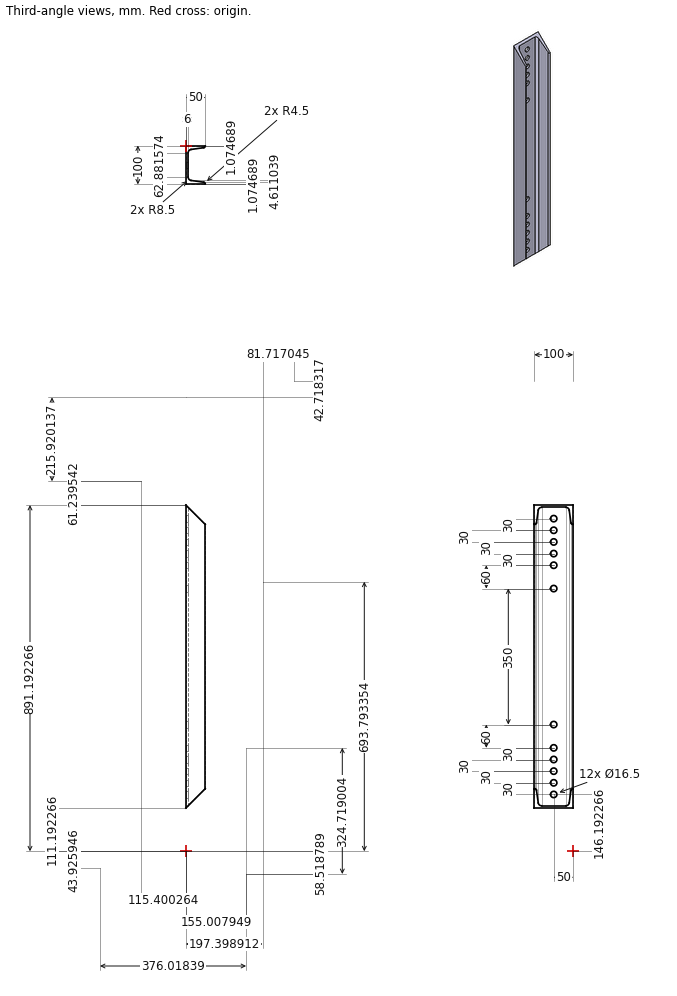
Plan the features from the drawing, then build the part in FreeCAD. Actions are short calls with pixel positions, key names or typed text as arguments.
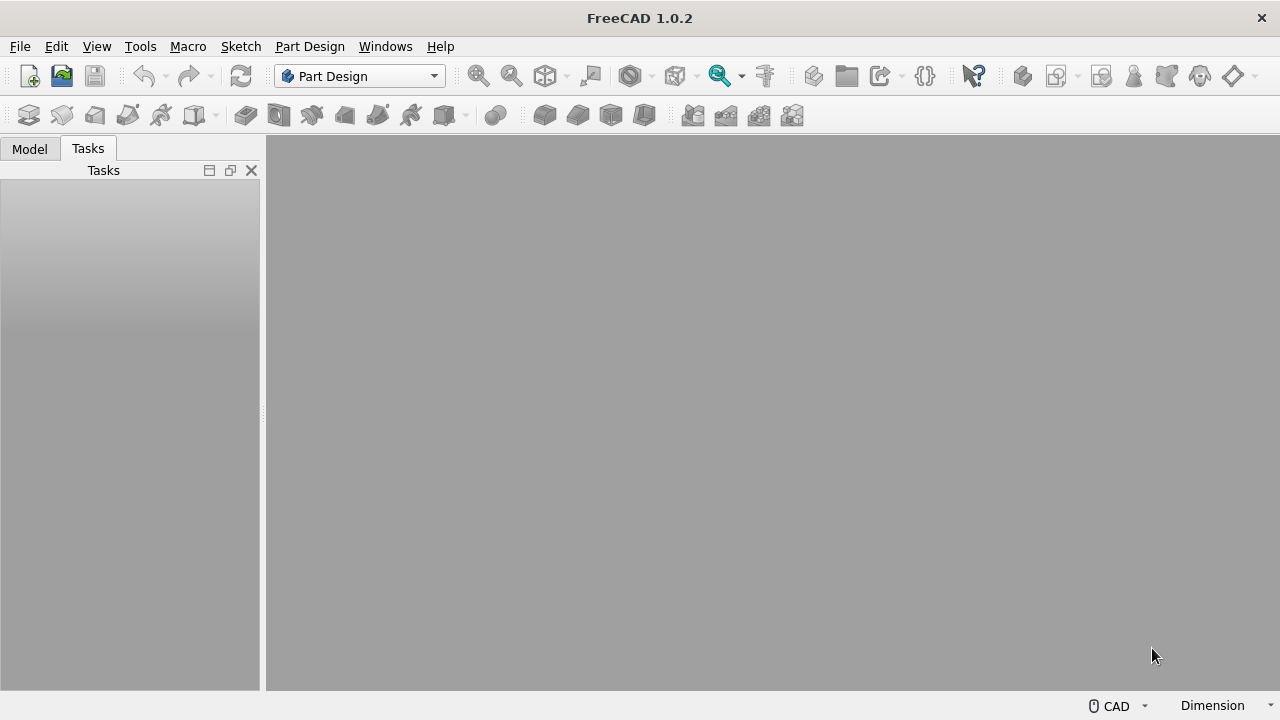
click(29, 76)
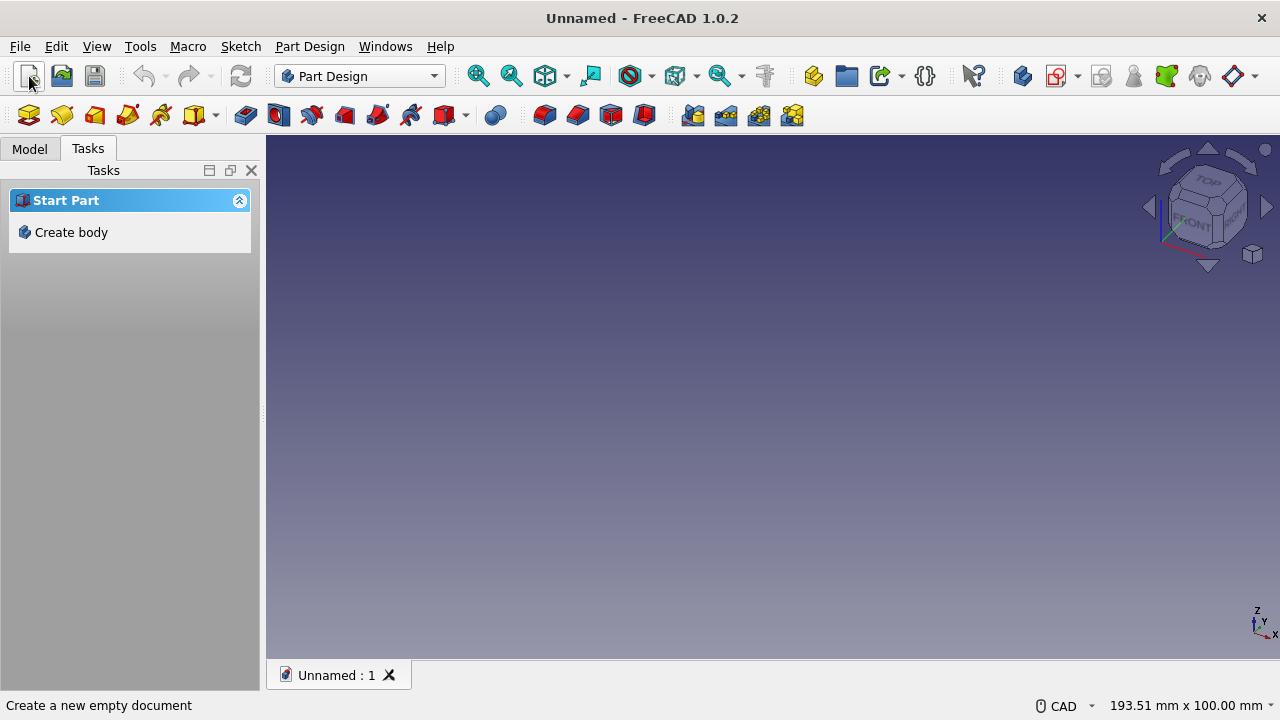
click(1056, 76)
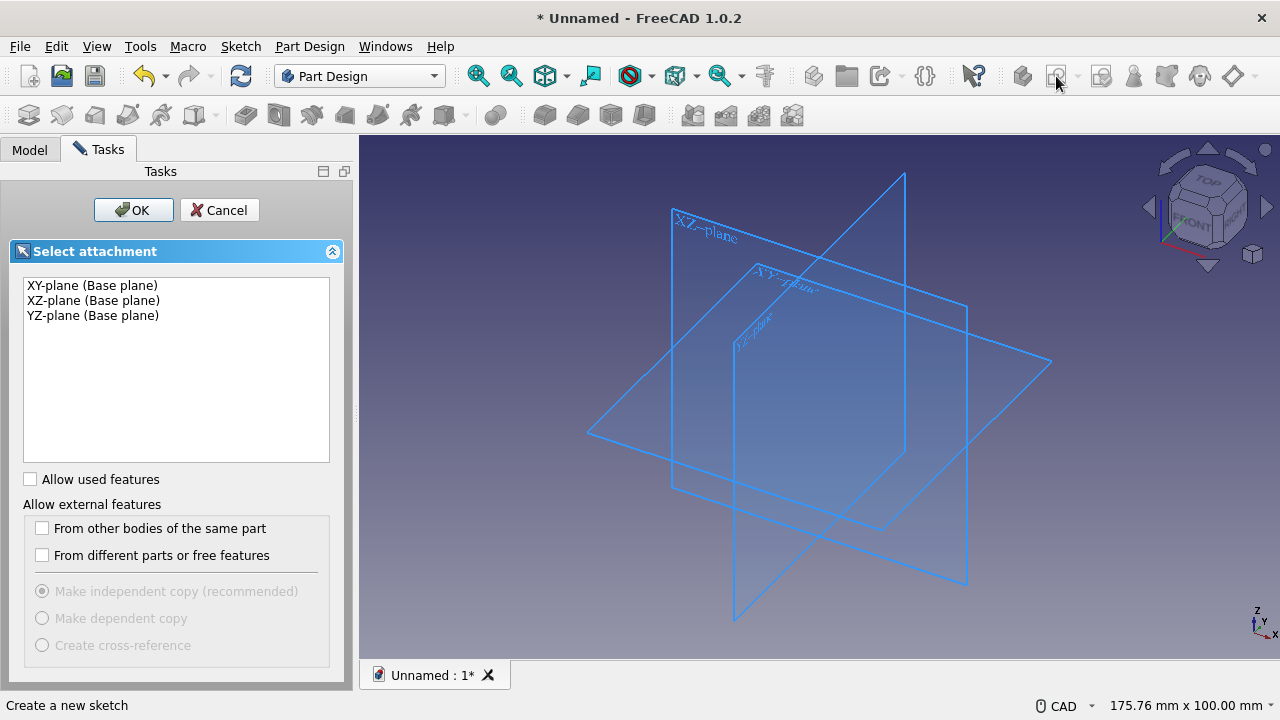
click(84, 286)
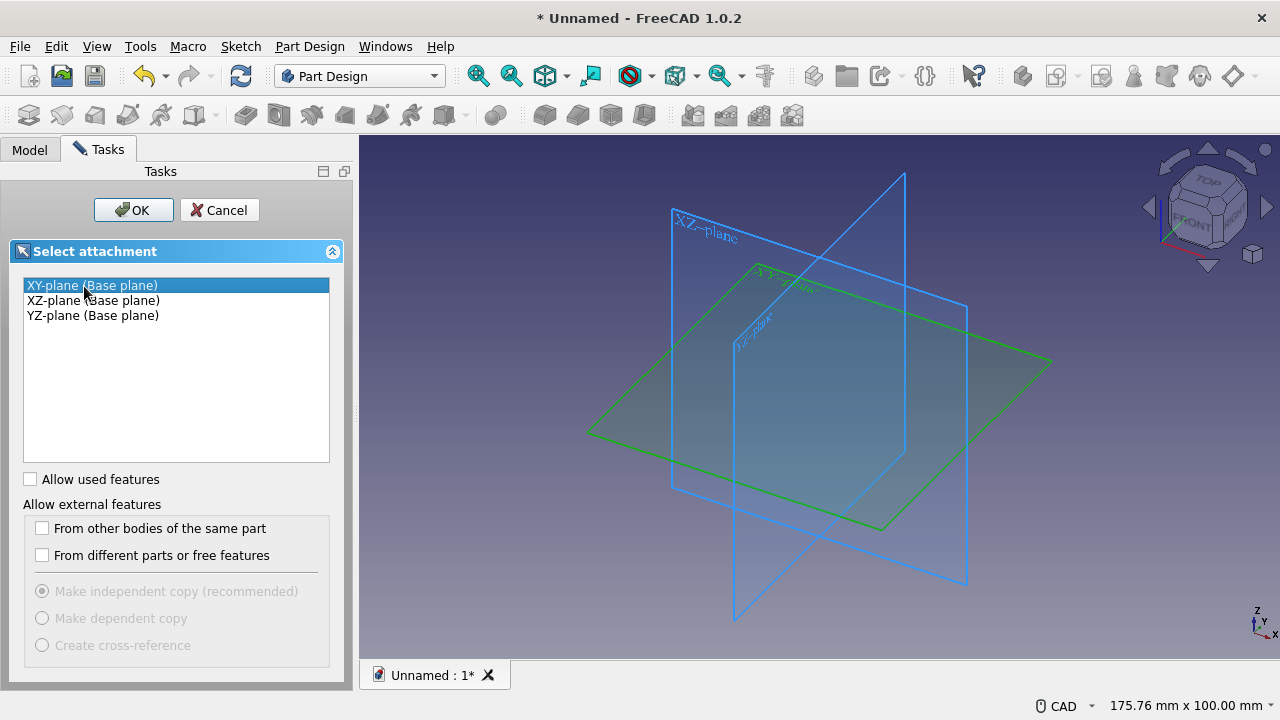
click(134, 210)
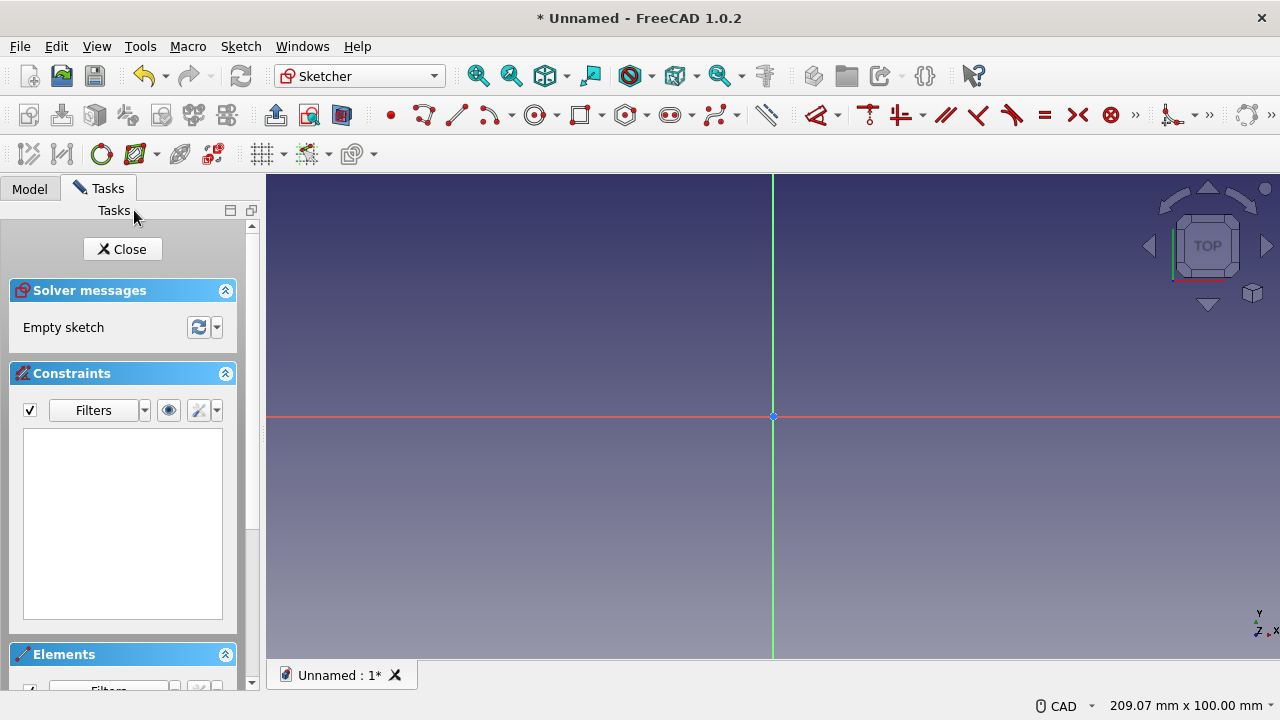
scroll(474, 202, down, 3)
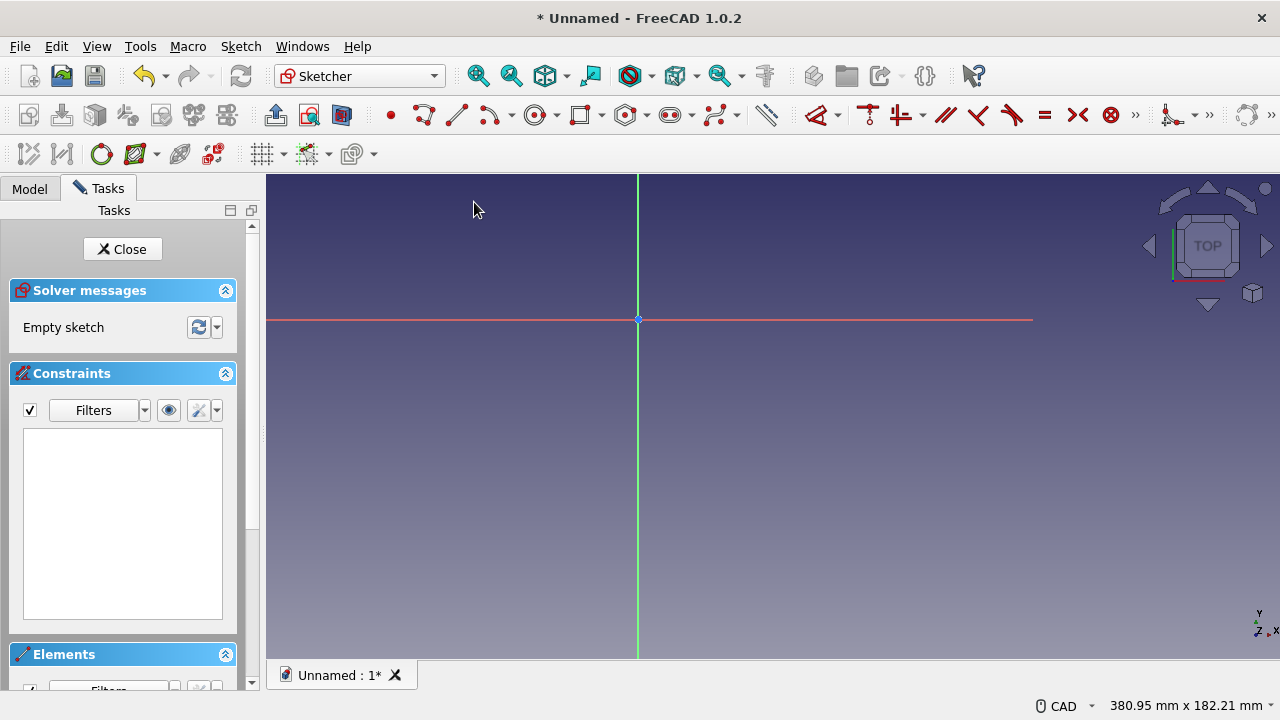
click(457, 116)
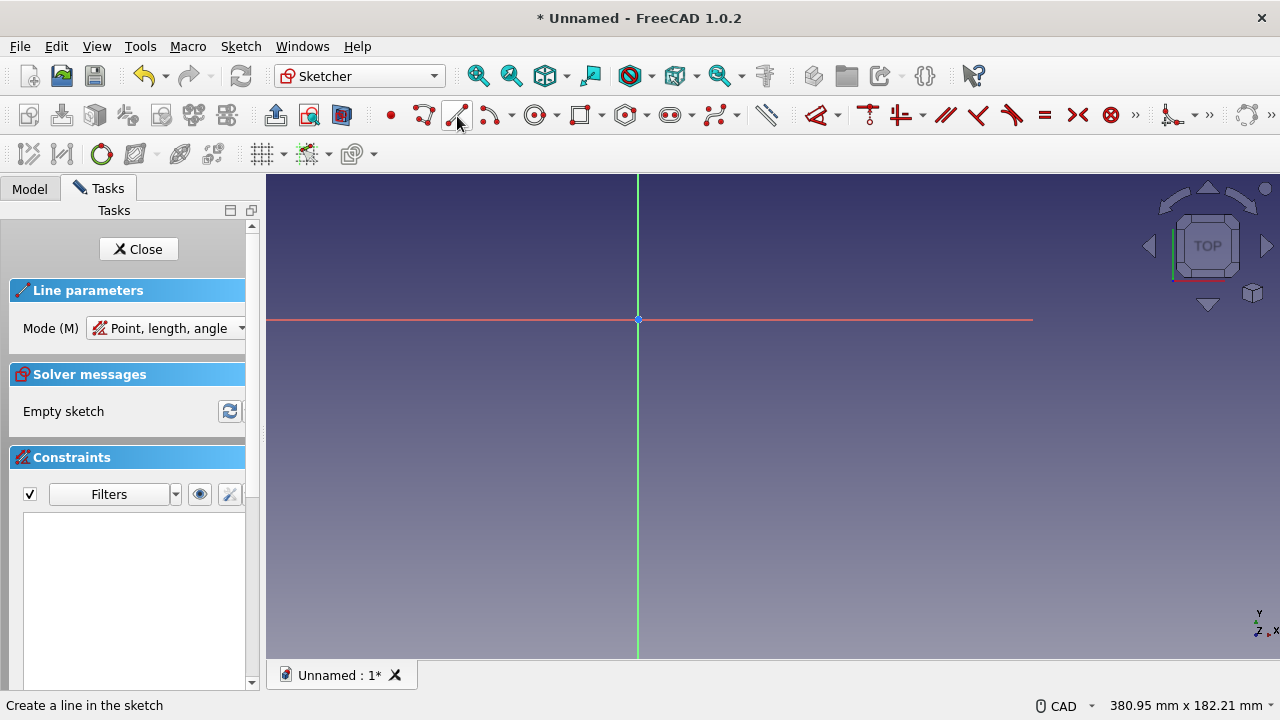
click(761, 571)
click(674, 559)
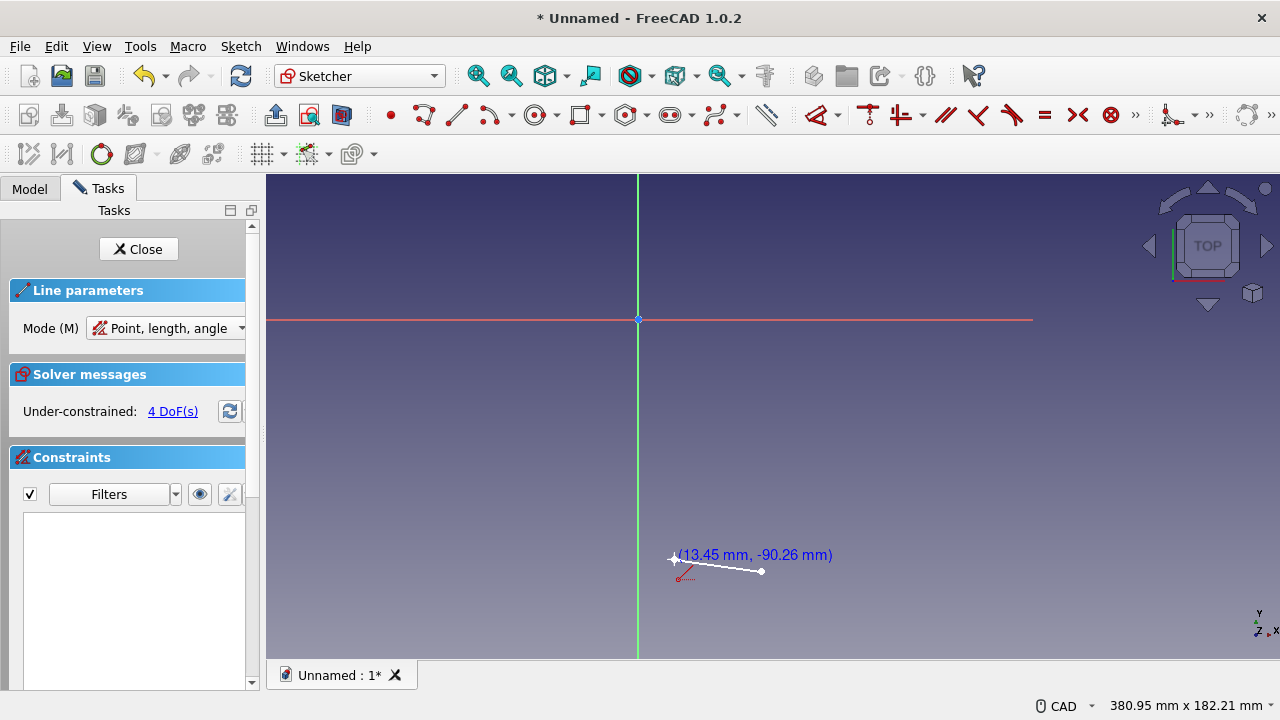
click(654, 537)
click(654, 369)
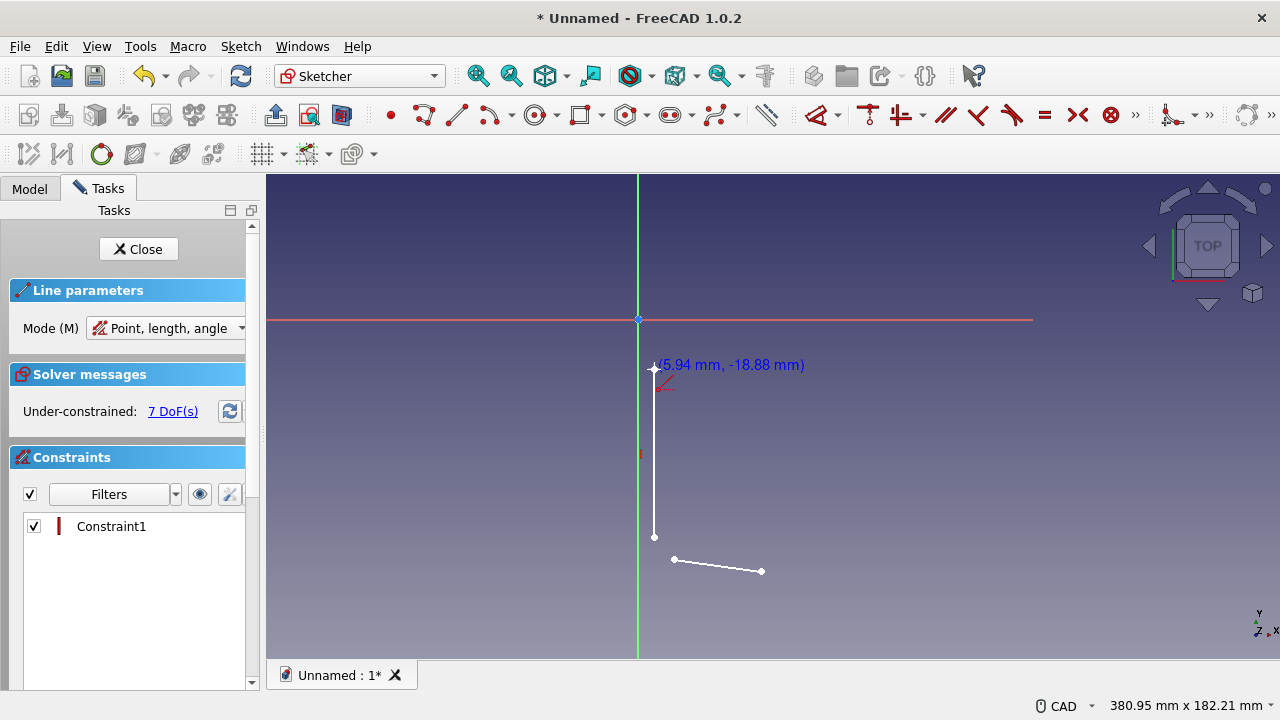
click(674, 347)
click(761, 334)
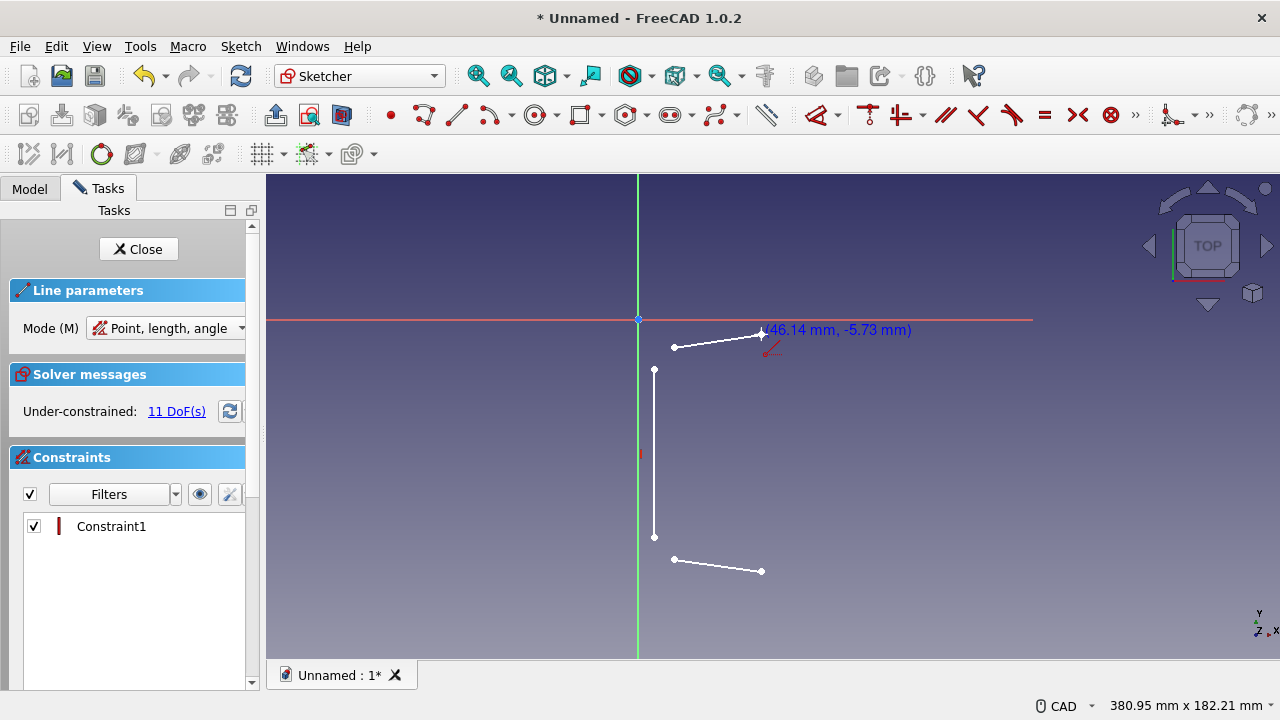
click(424, 116)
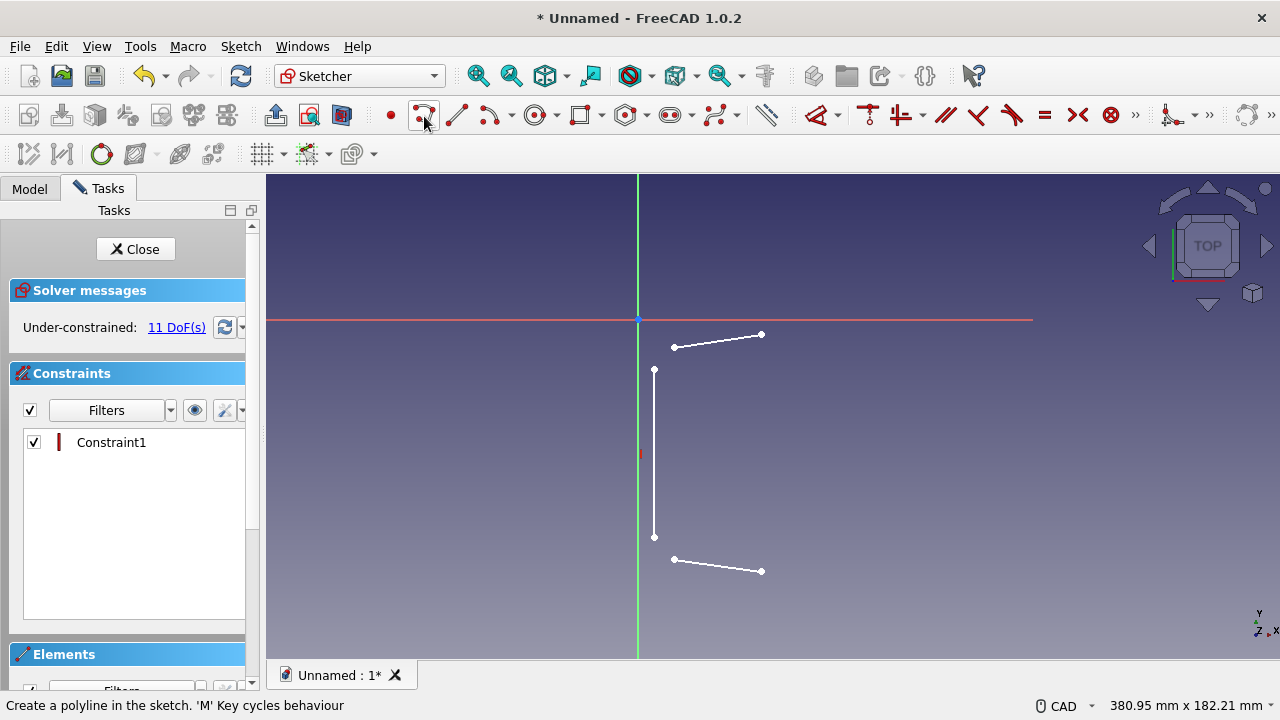
scroll(771, 323, up, 9)